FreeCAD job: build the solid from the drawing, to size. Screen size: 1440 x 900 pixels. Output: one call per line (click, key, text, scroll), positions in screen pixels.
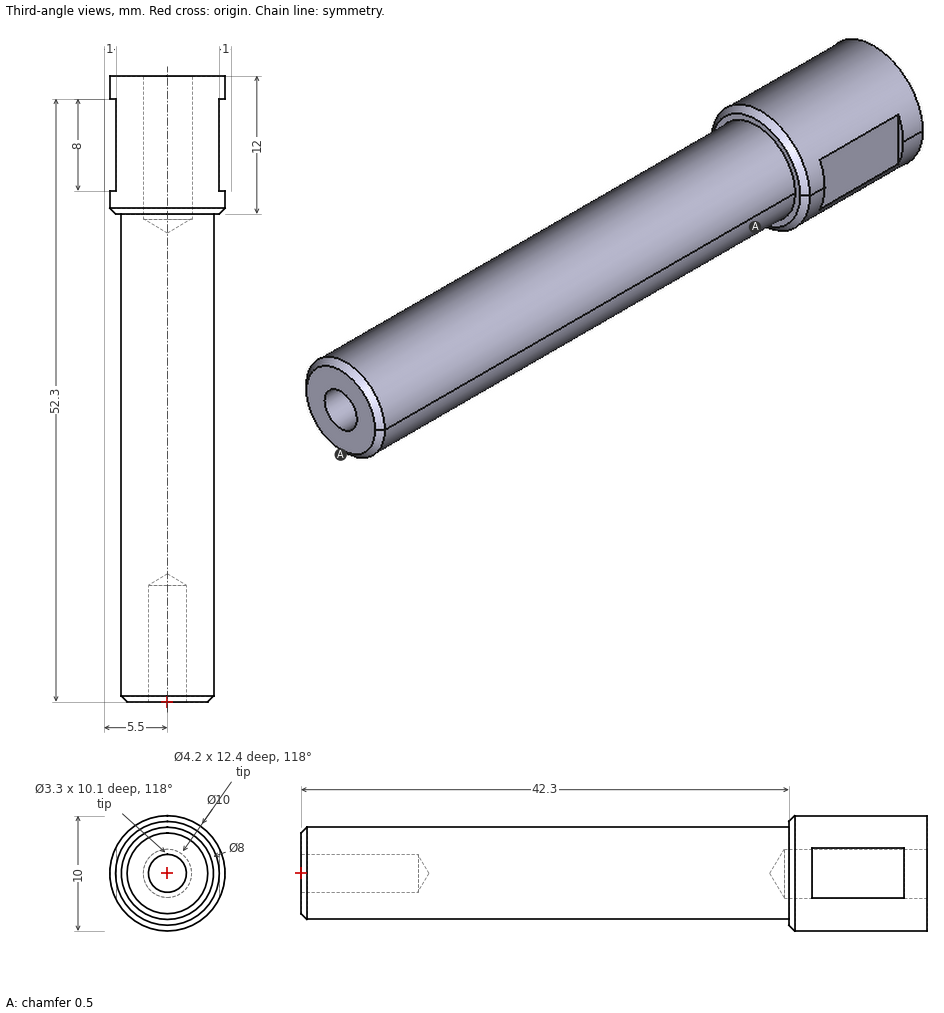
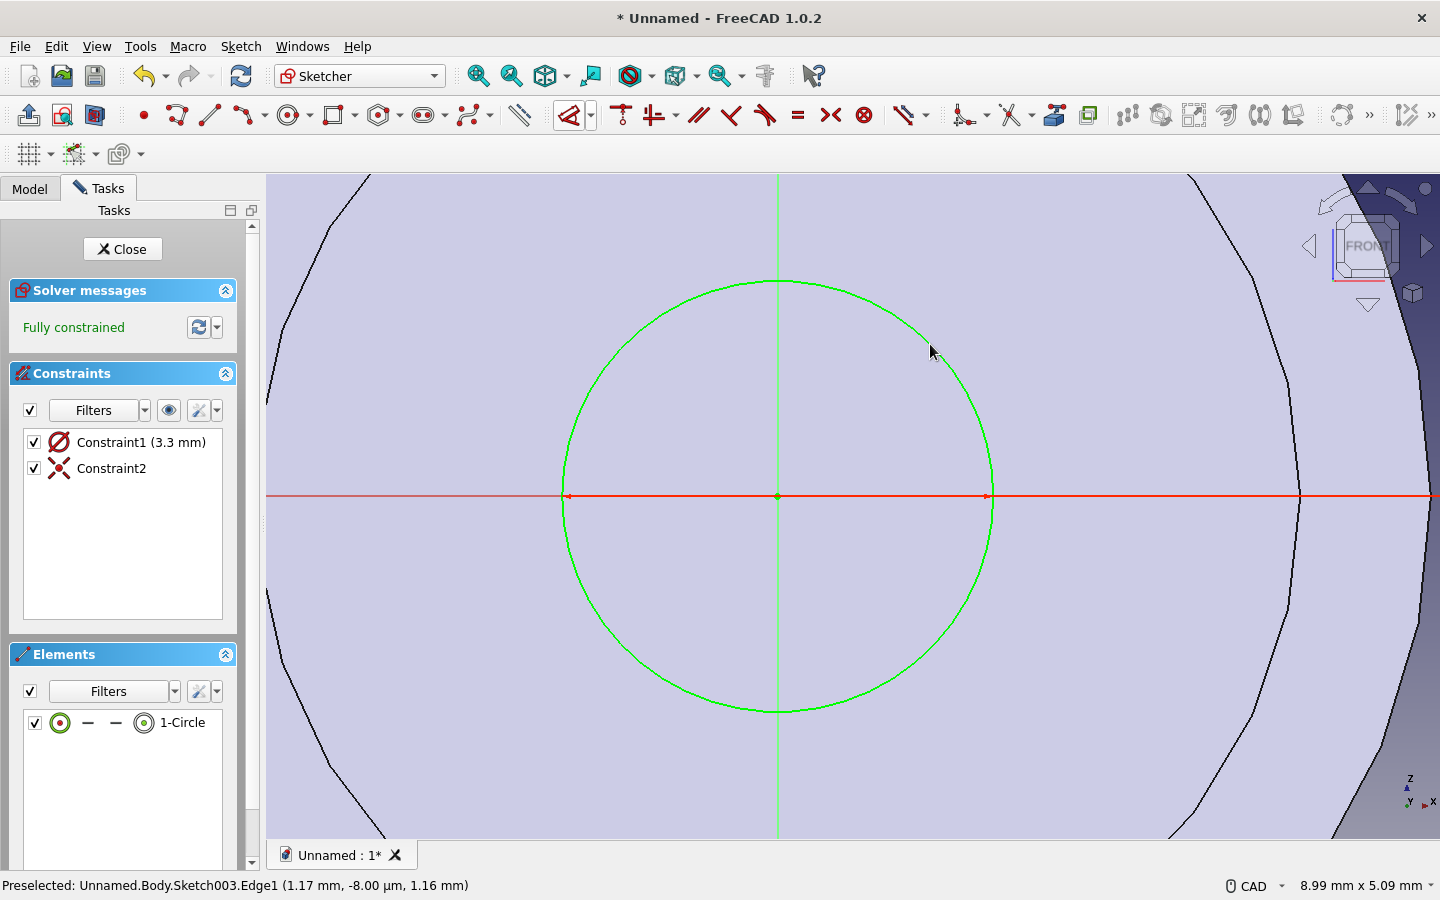
click(123, 249)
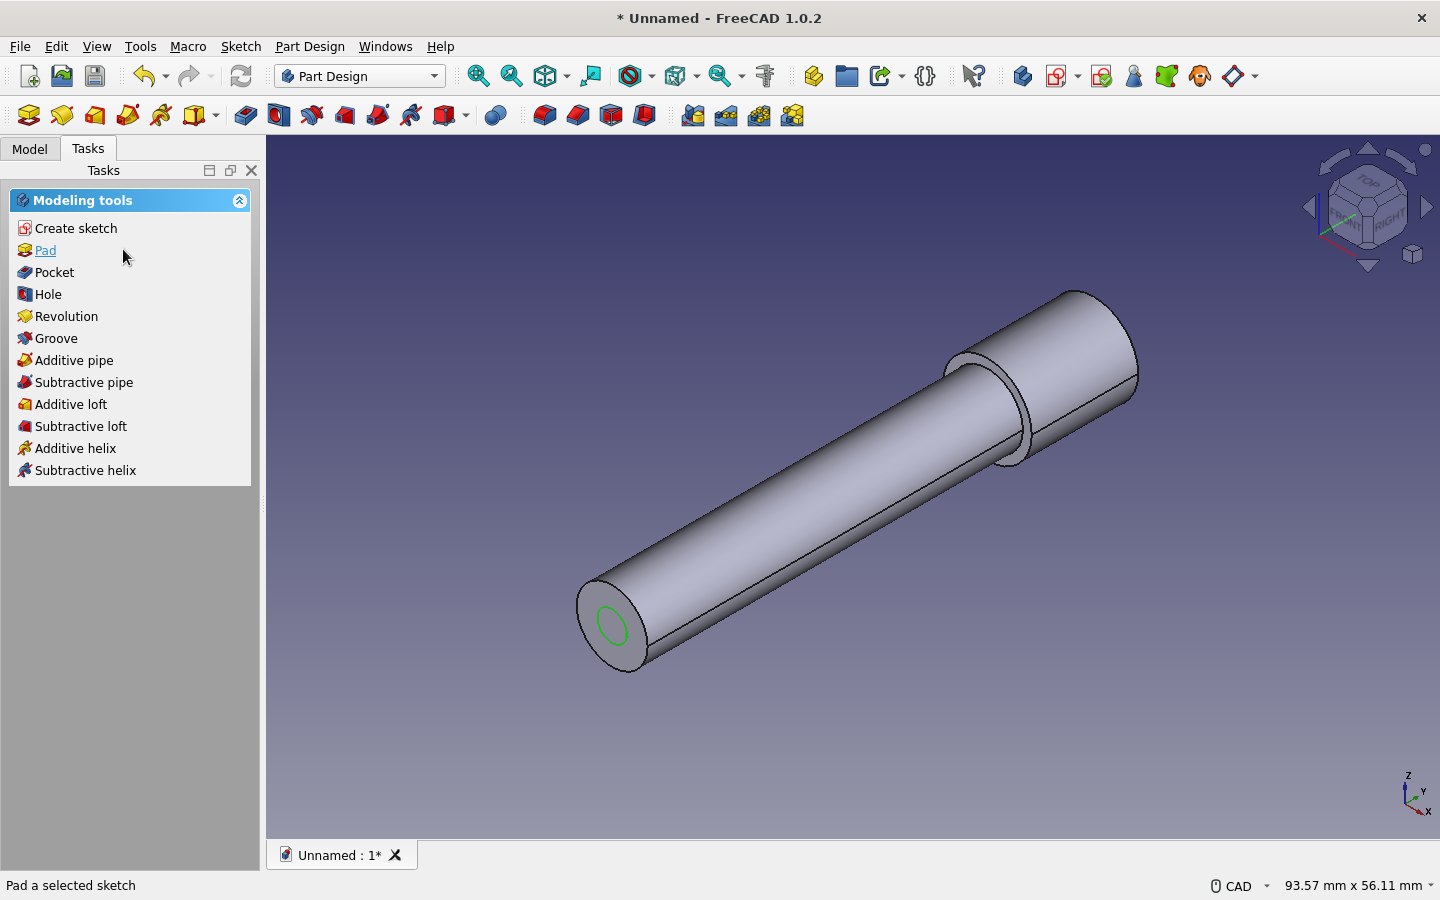
click(279, 116)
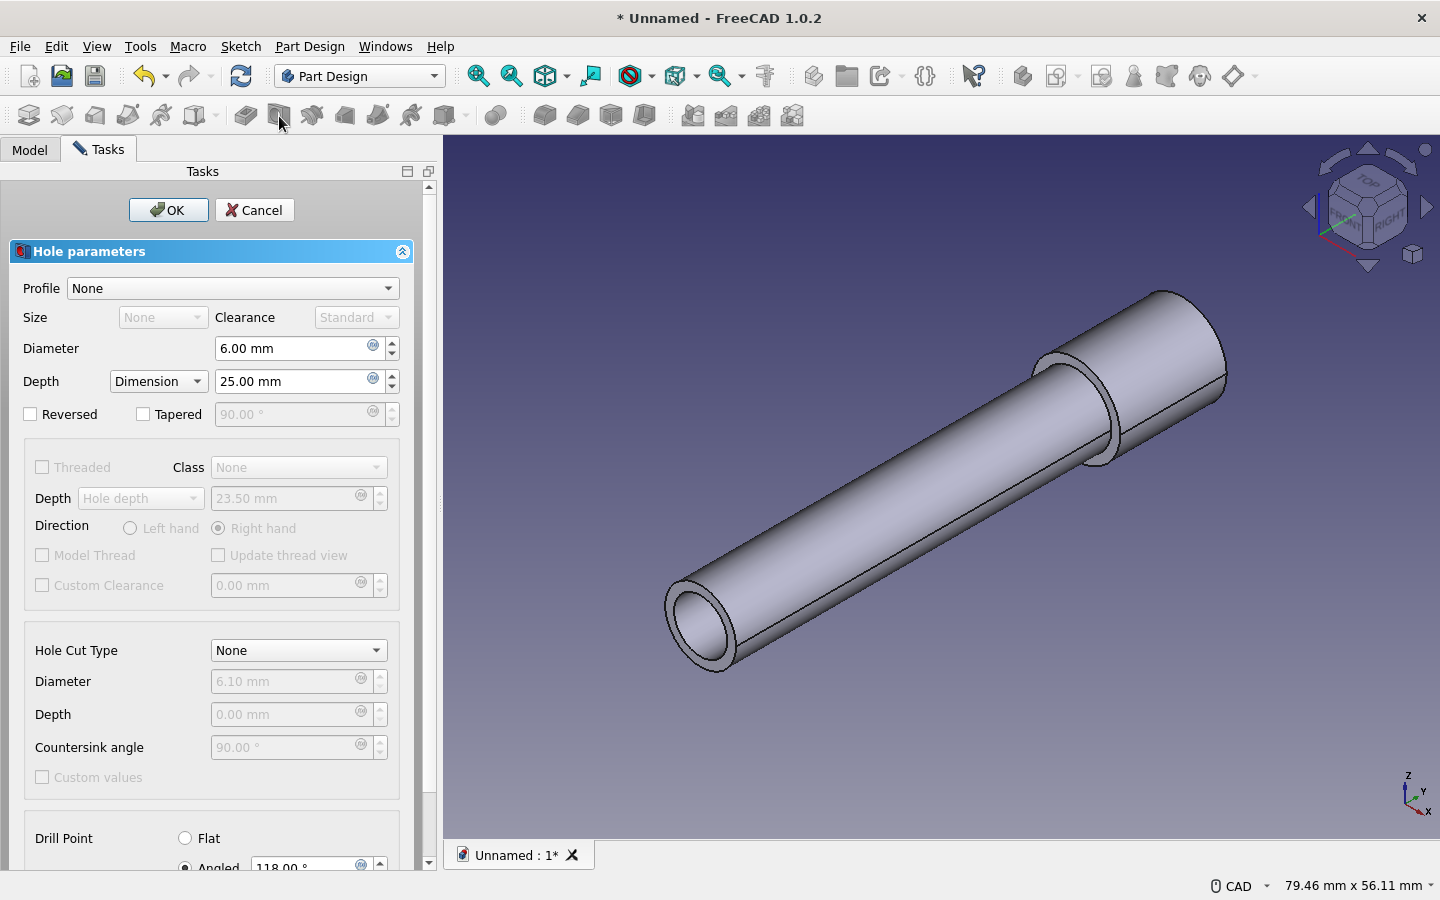
triple_click(300, 348)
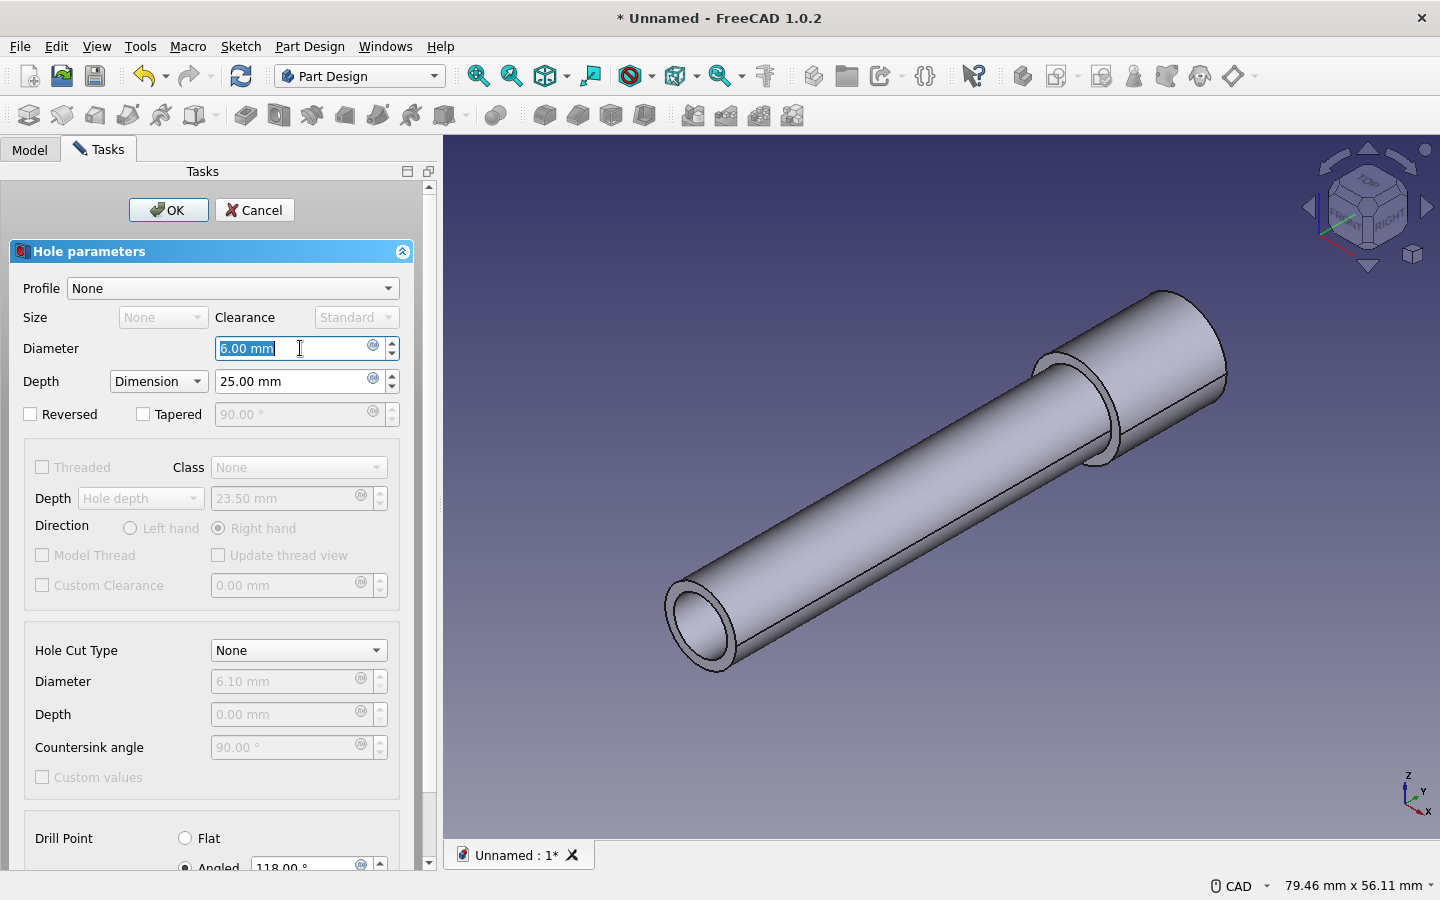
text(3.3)
key(Tab)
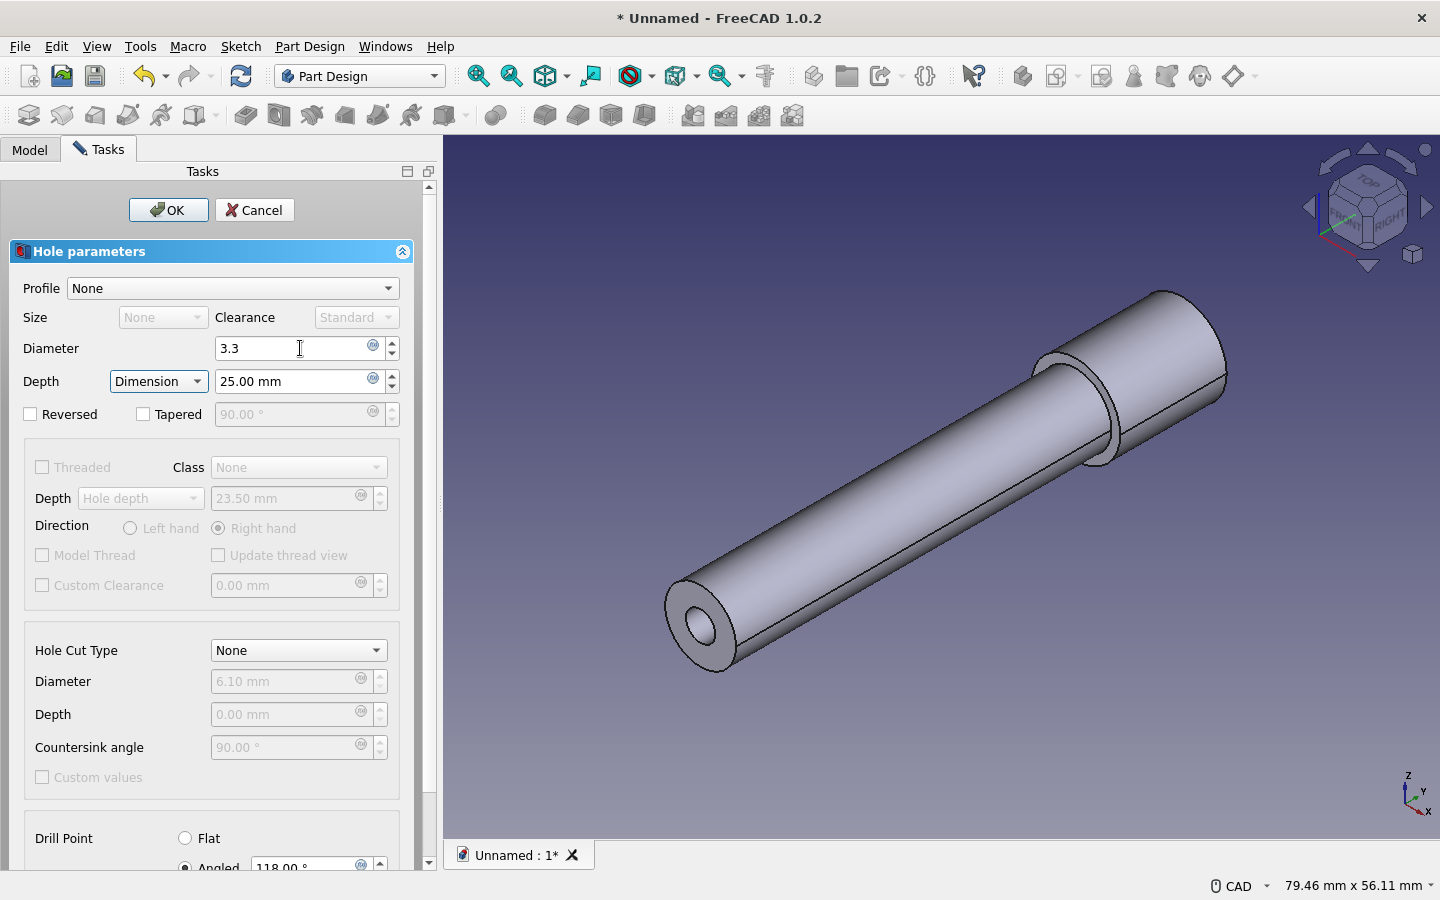
triple_click(300, 382)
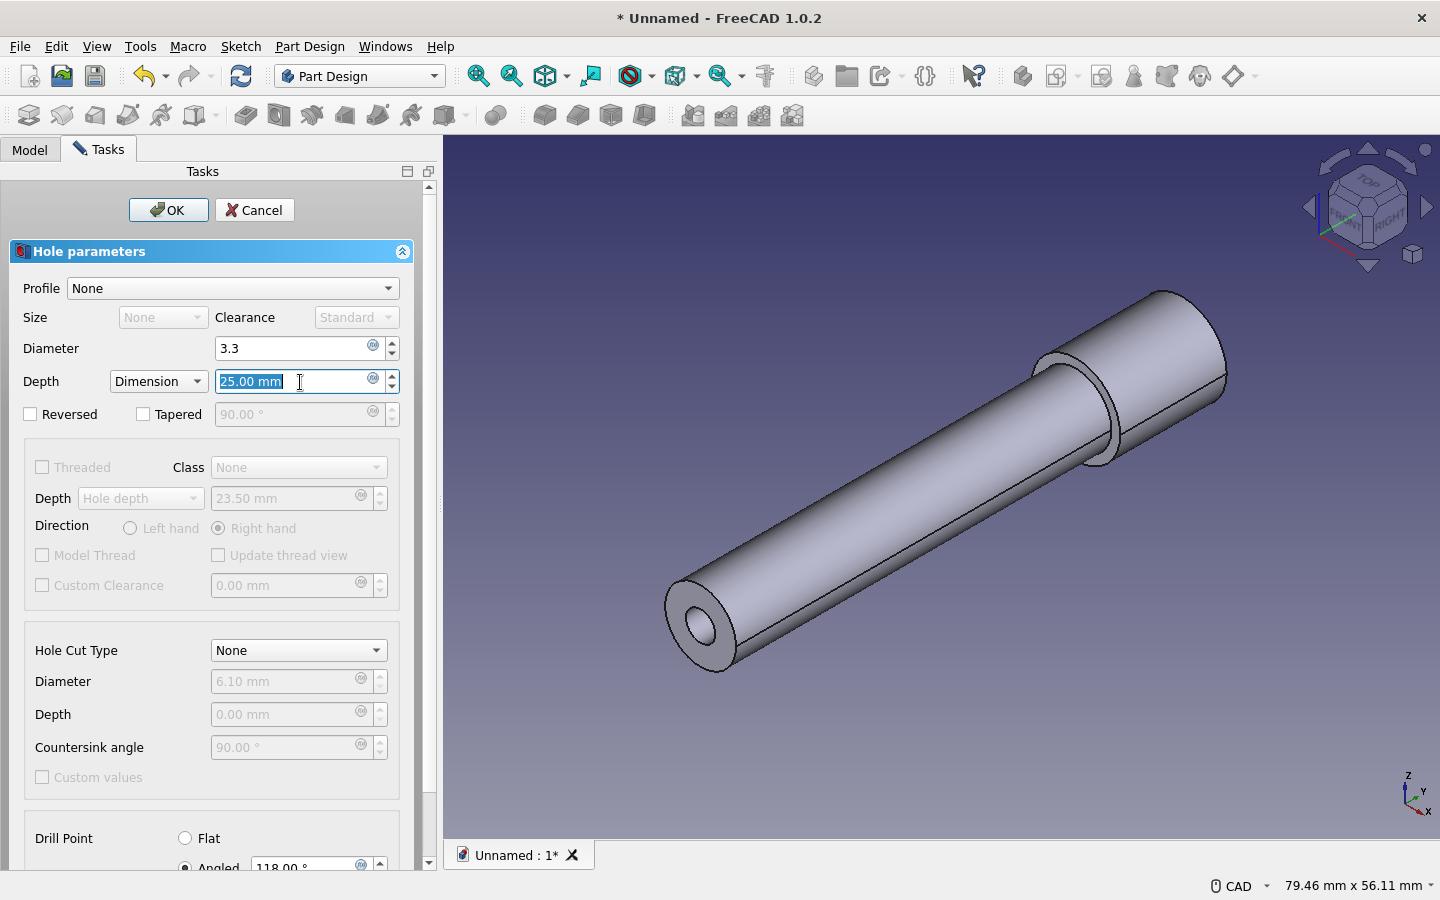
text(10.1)
key(Tab)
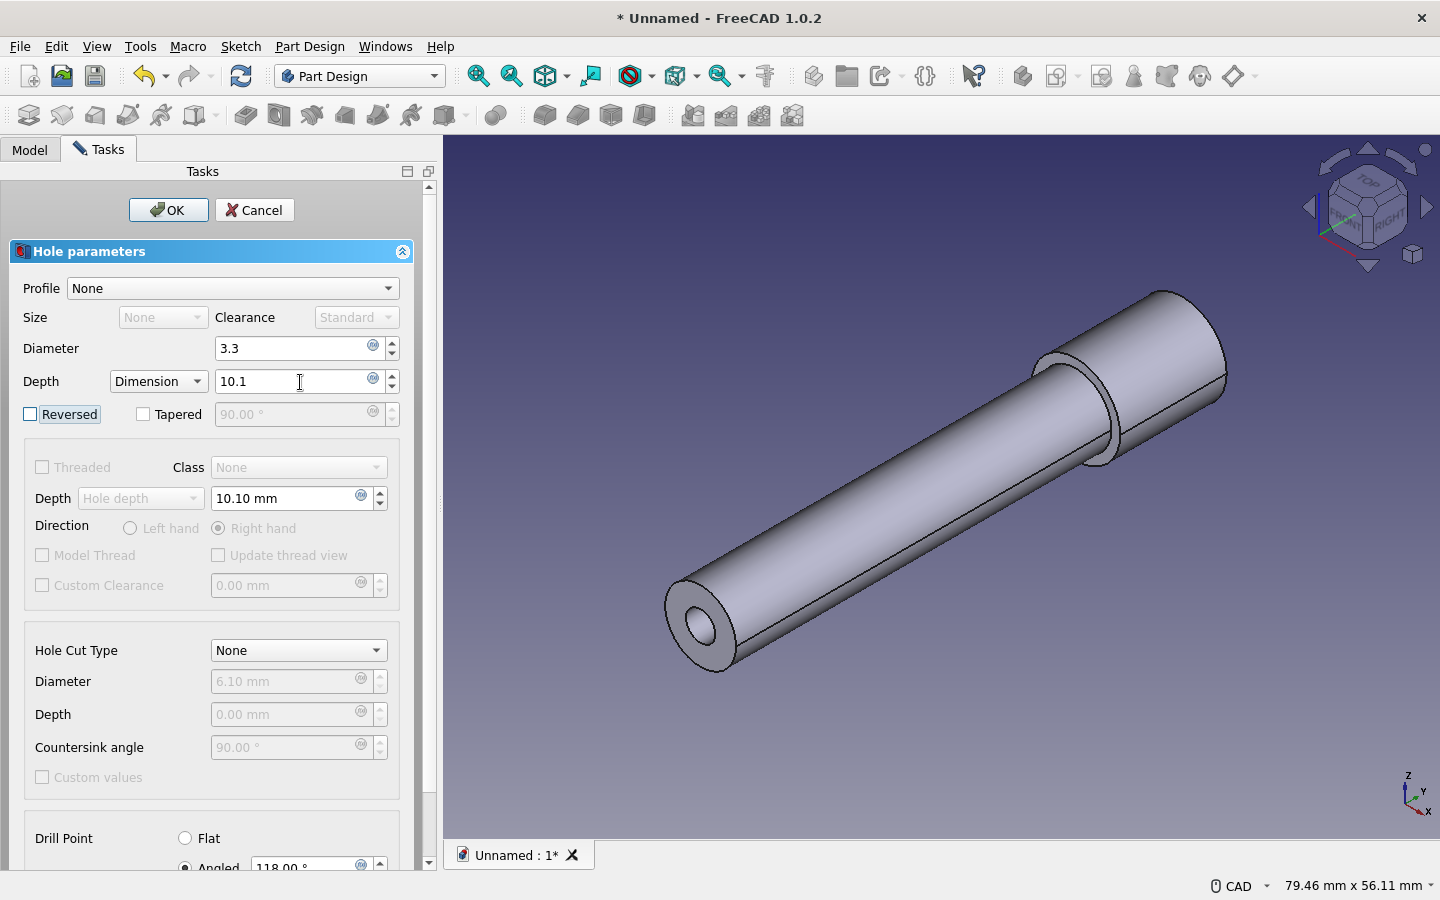
click(169, 210)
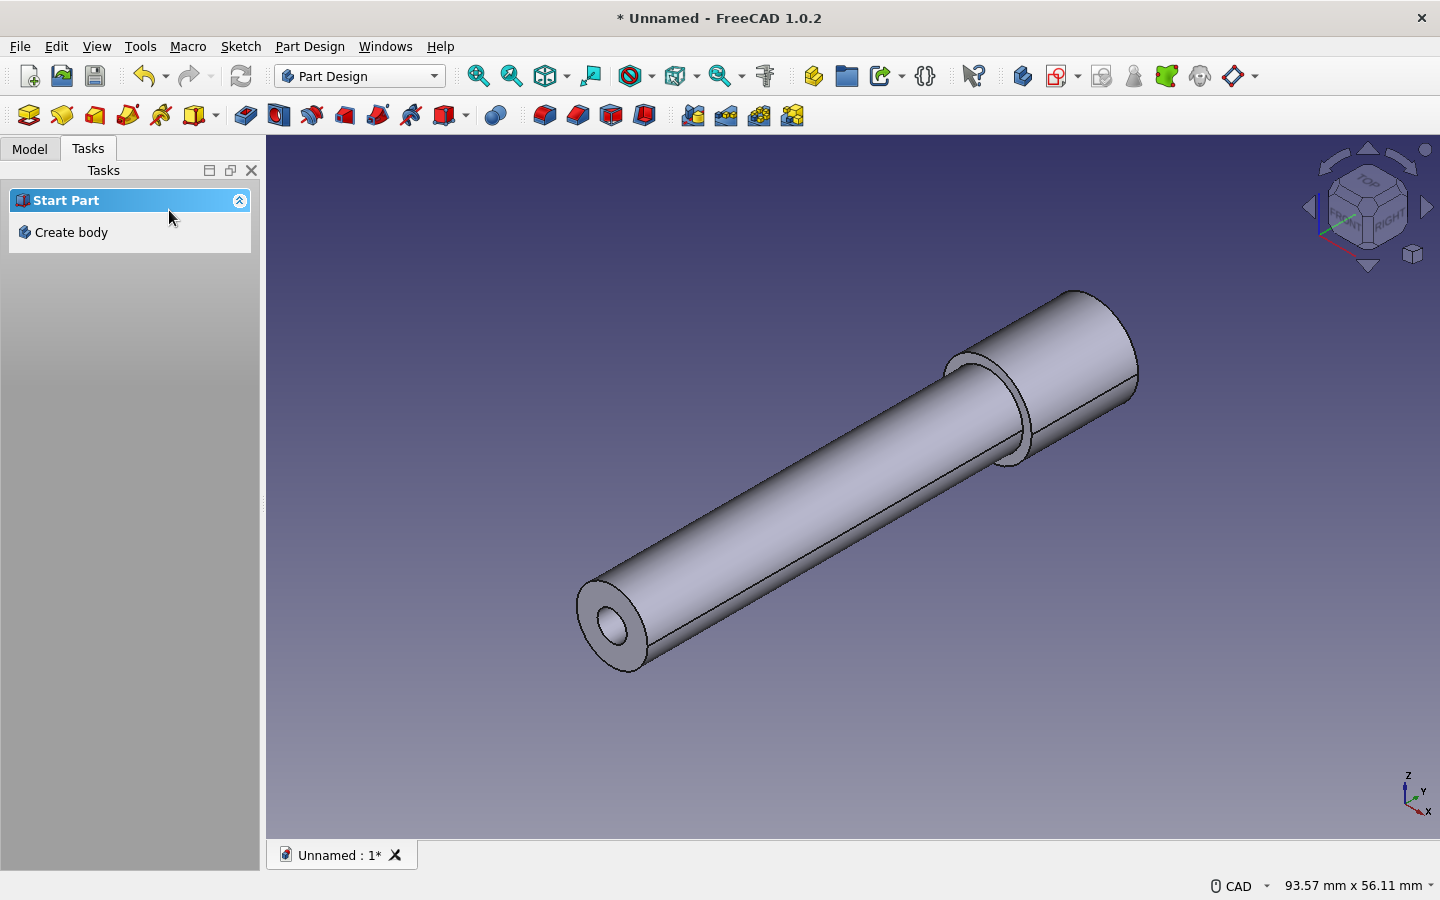
click(1056, 76)